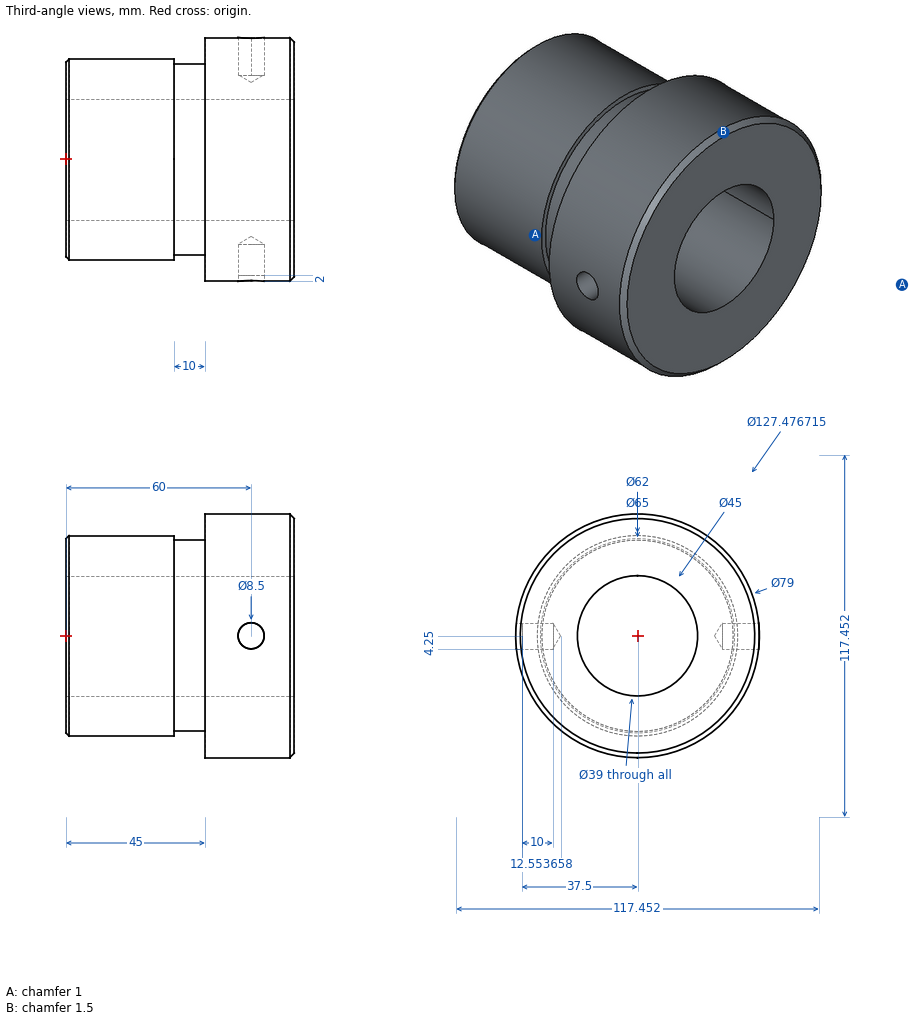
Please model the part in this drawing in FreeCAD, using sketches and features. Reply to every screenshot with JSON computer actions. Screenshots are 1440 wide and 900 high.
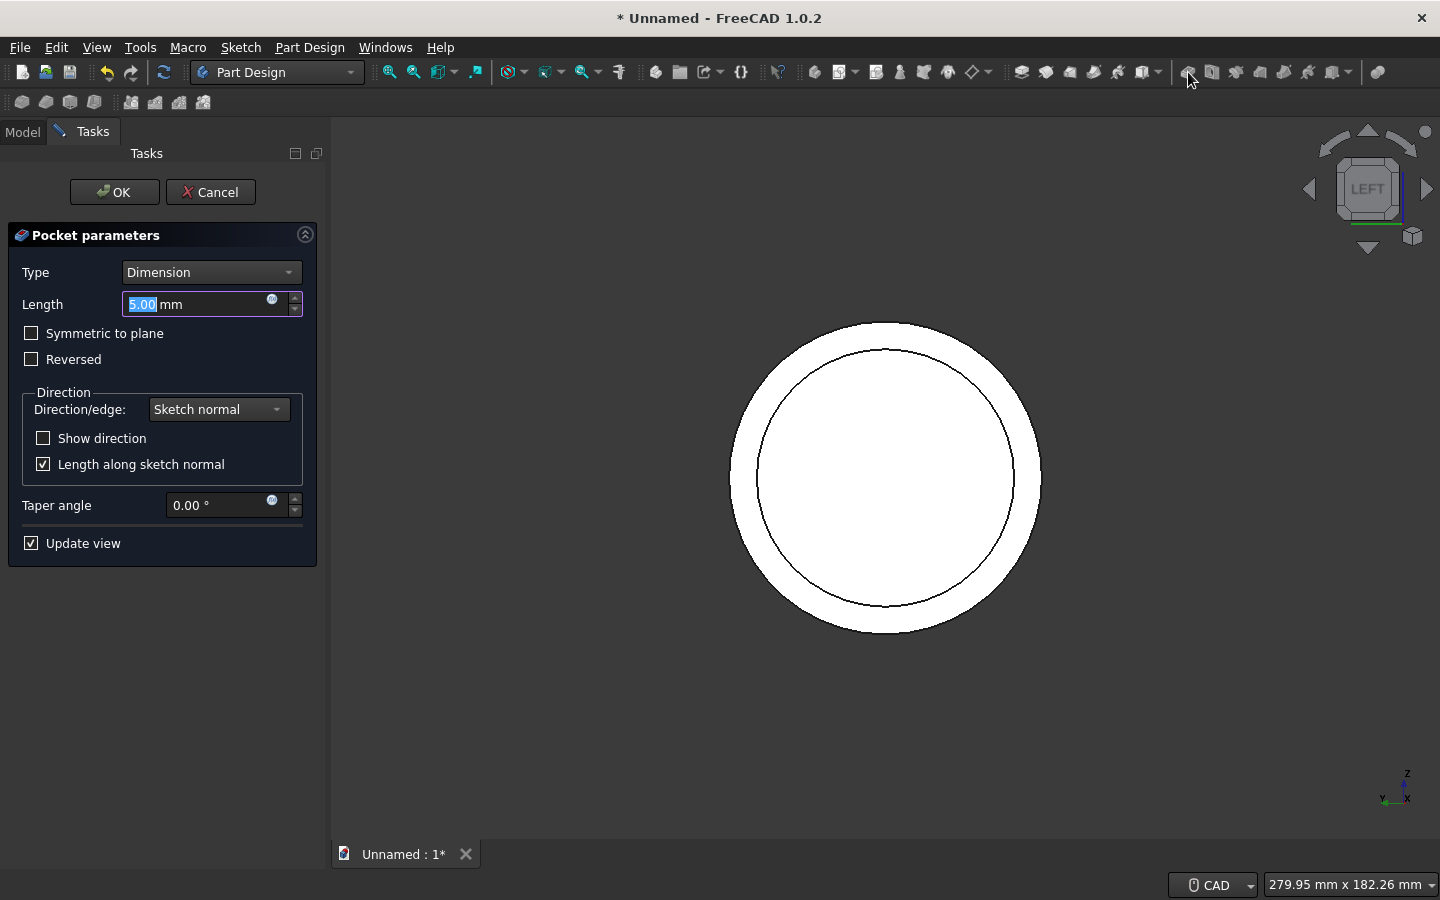
{"action": "type", "text": "45"}
{"action": "key", "text": "Tab"}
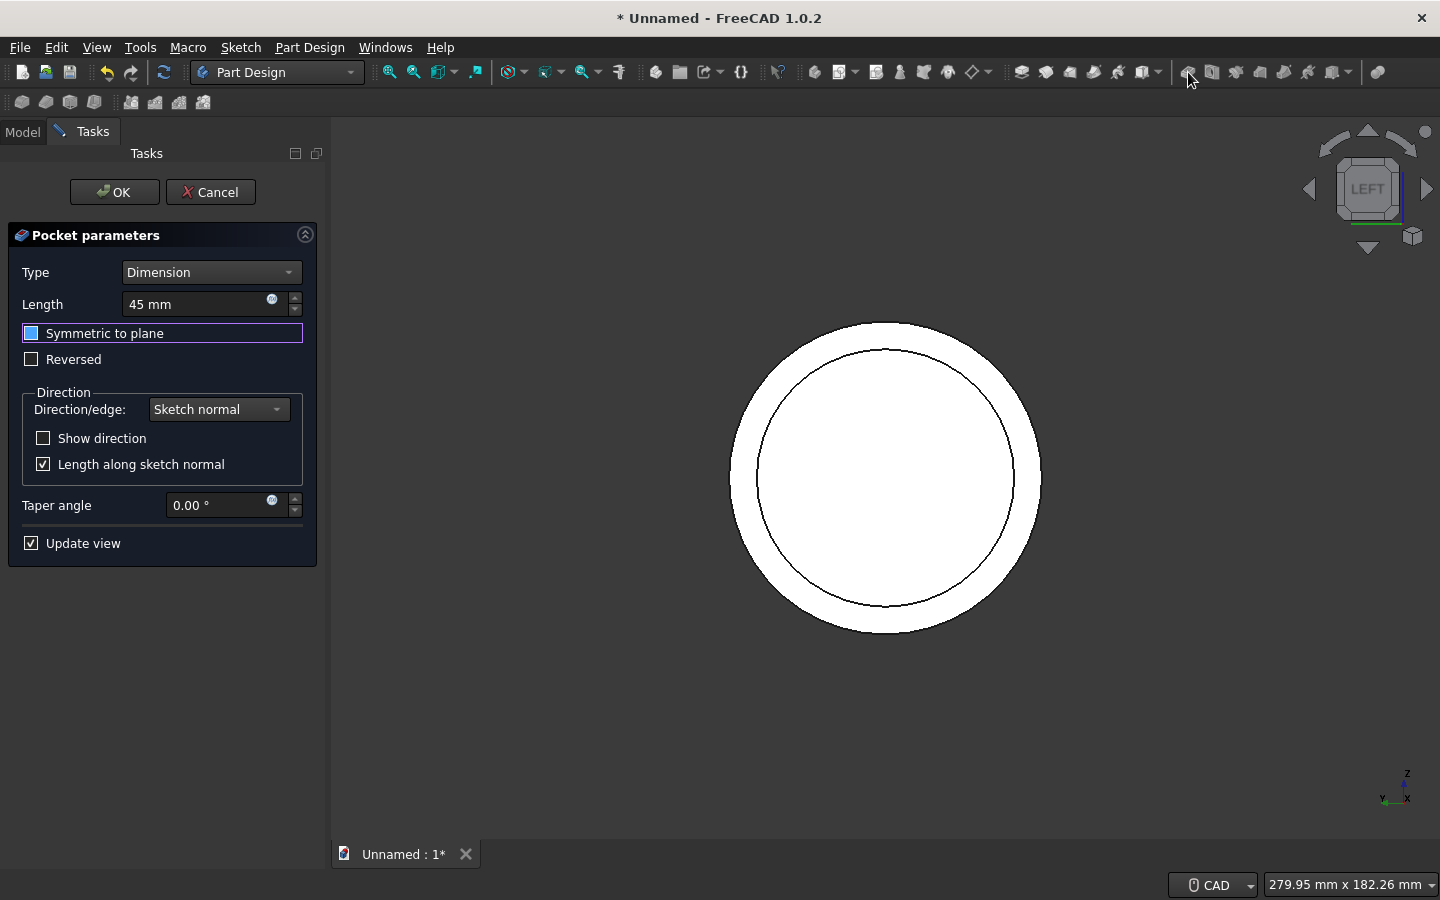
{"action": "left_click", "coordinate": [115, 192]}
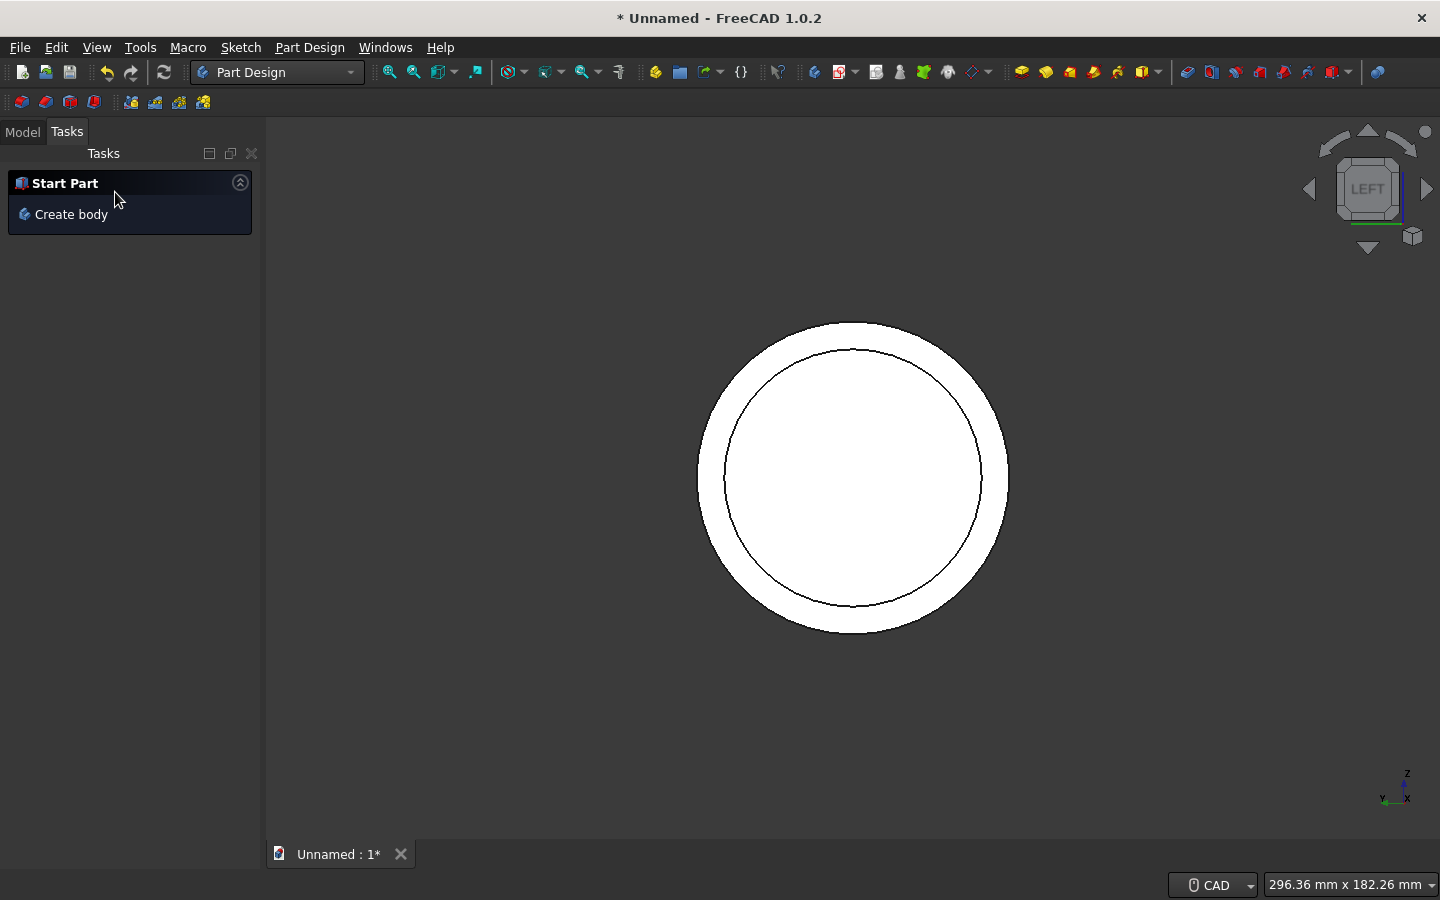
{"action": "key", "text": "v f"}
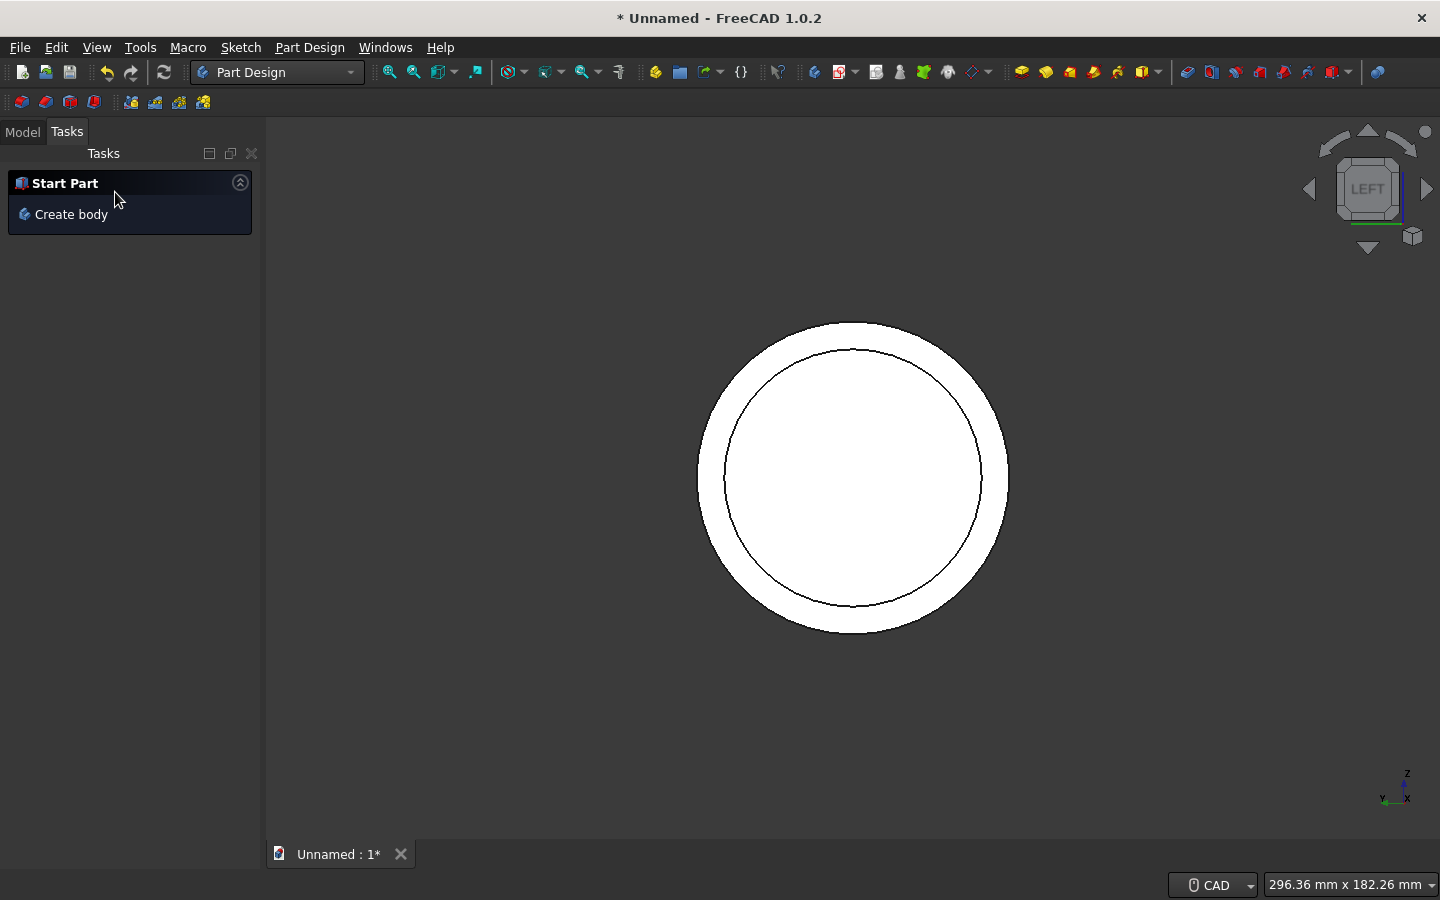
{"action": "left_click", "coordinate": [898, 343]}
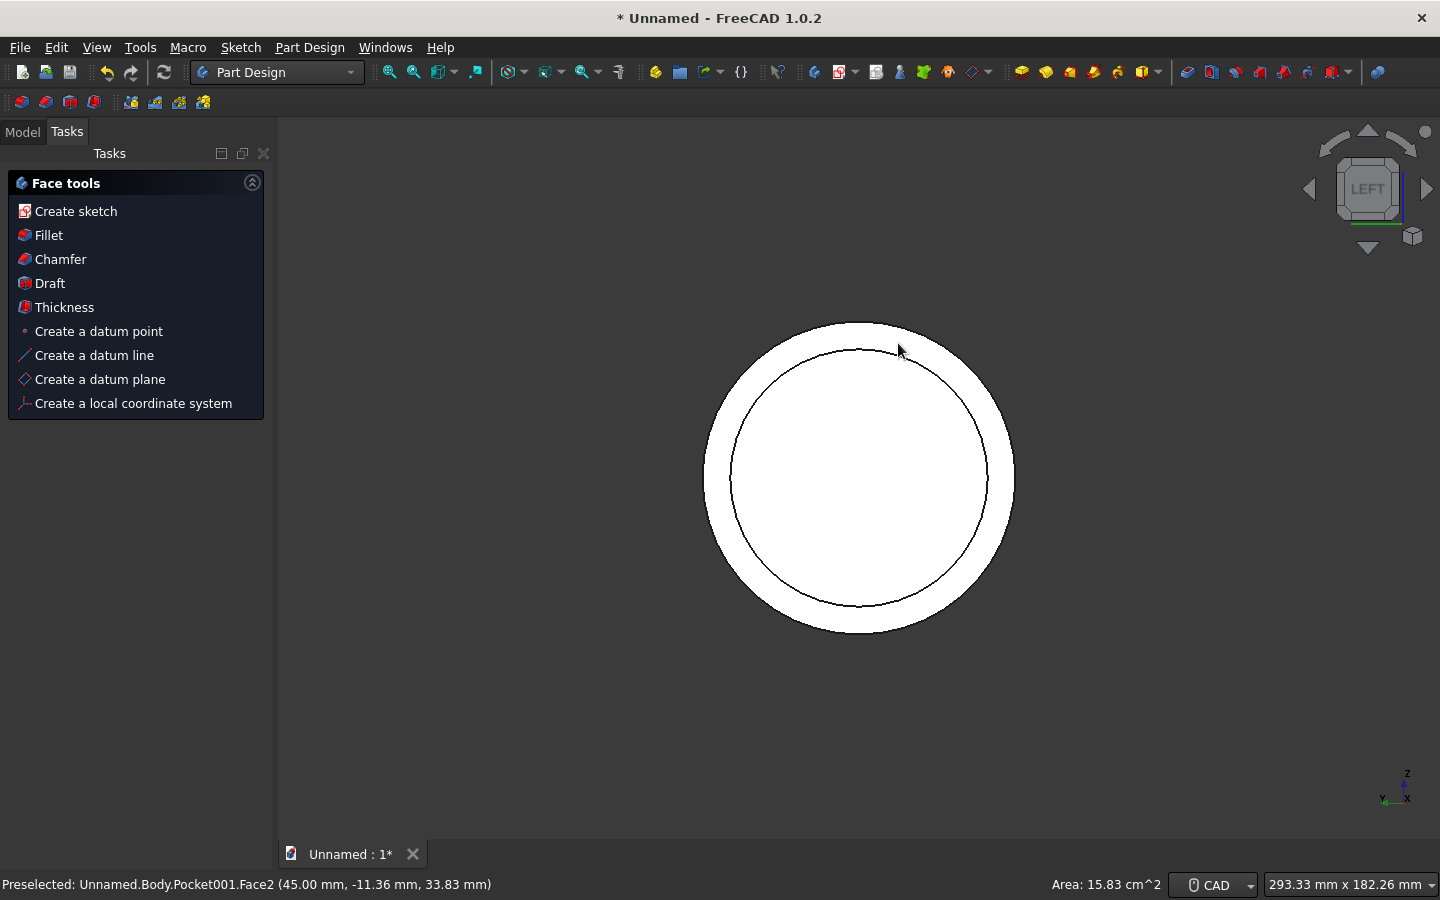
{"action": "left_click", "coordinate": [840, 72]}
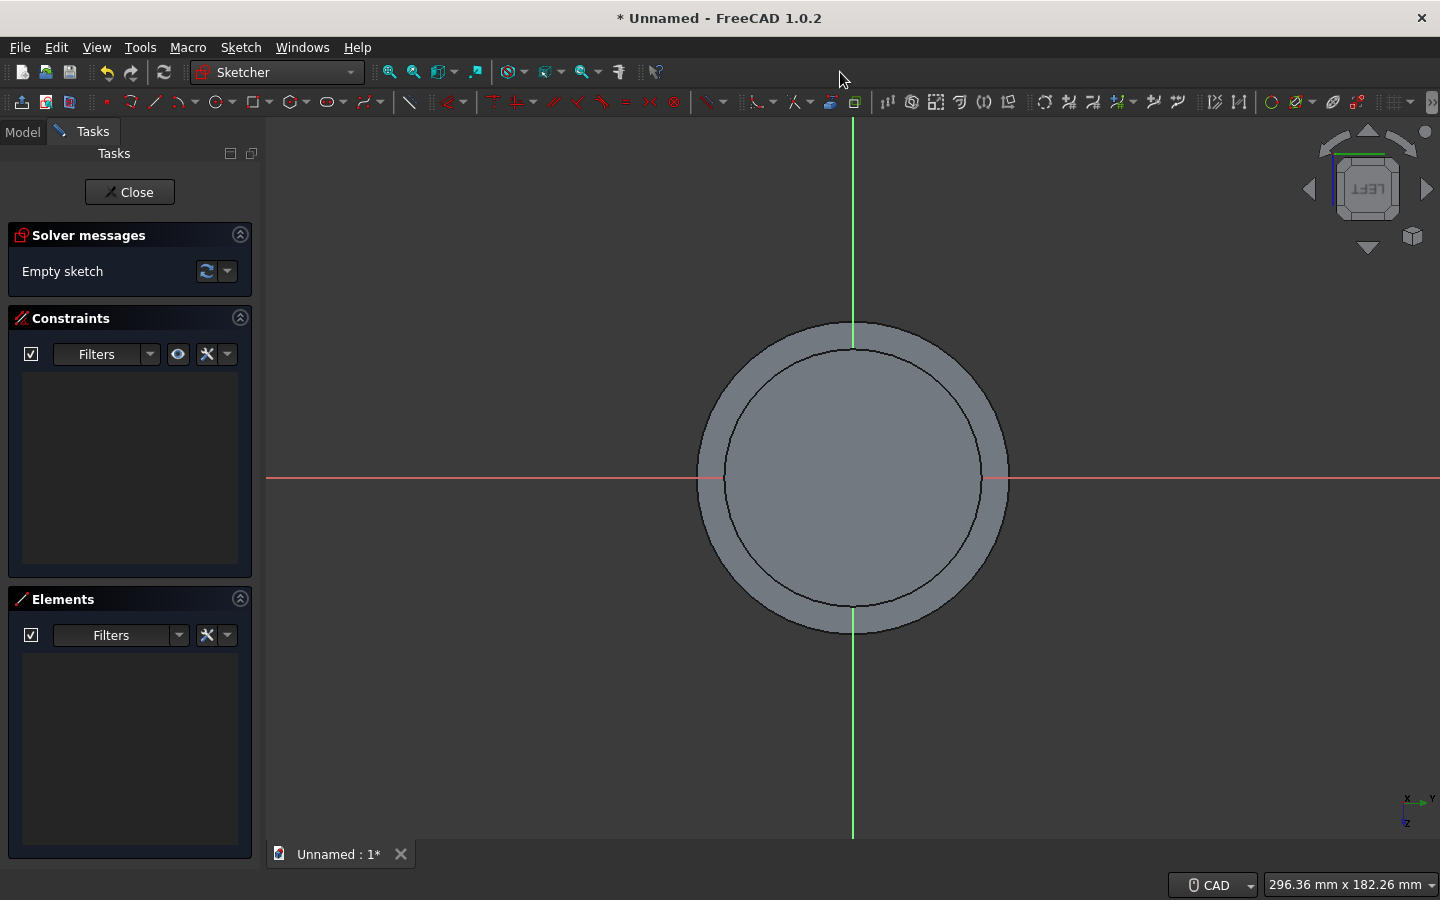
{"action": "key", "text": "g v"}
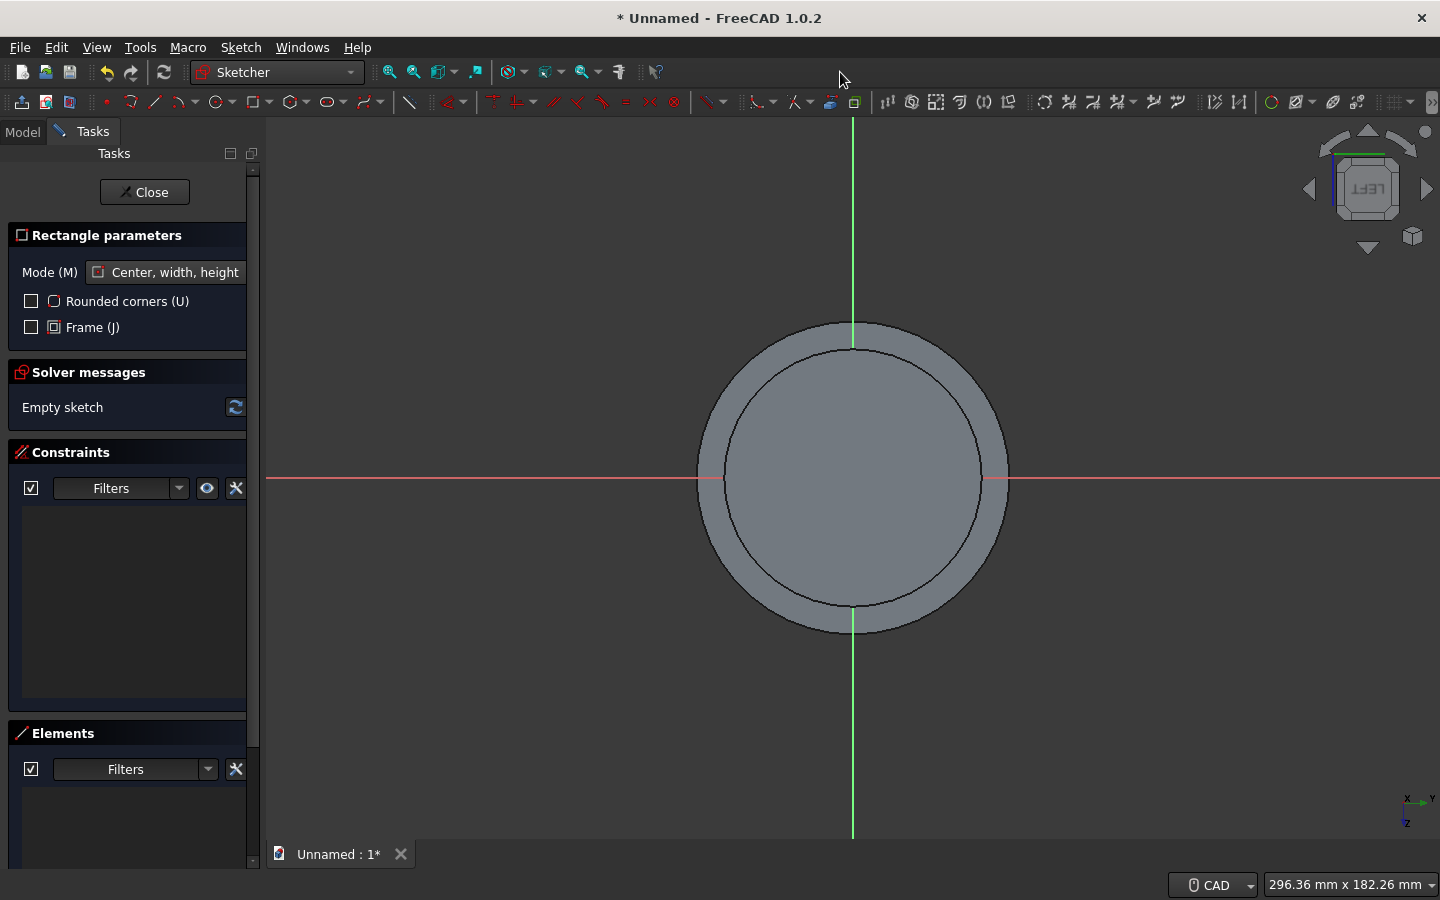
{"action": "left_click", "coordinate": [853, 478]}
{"action": "mouse_move", "coordinate": [1086, 245]}